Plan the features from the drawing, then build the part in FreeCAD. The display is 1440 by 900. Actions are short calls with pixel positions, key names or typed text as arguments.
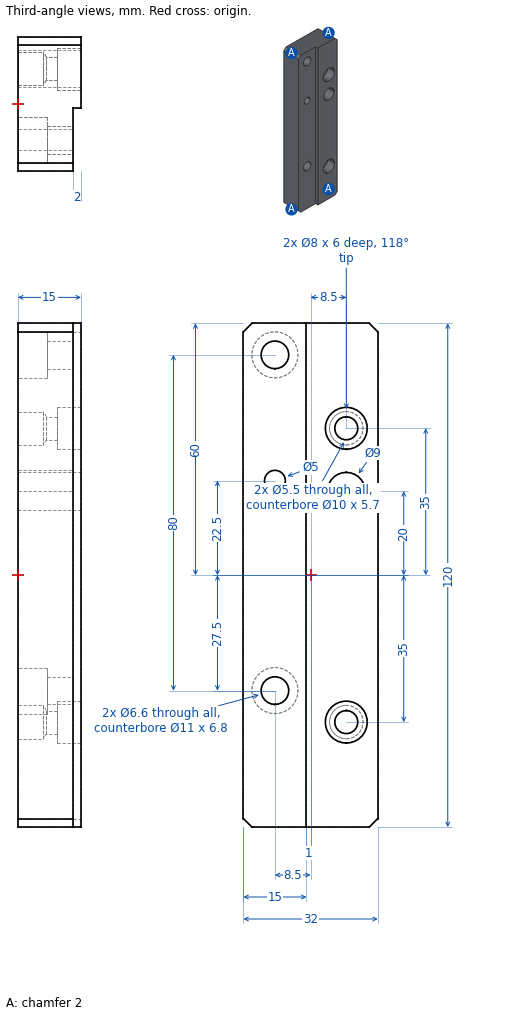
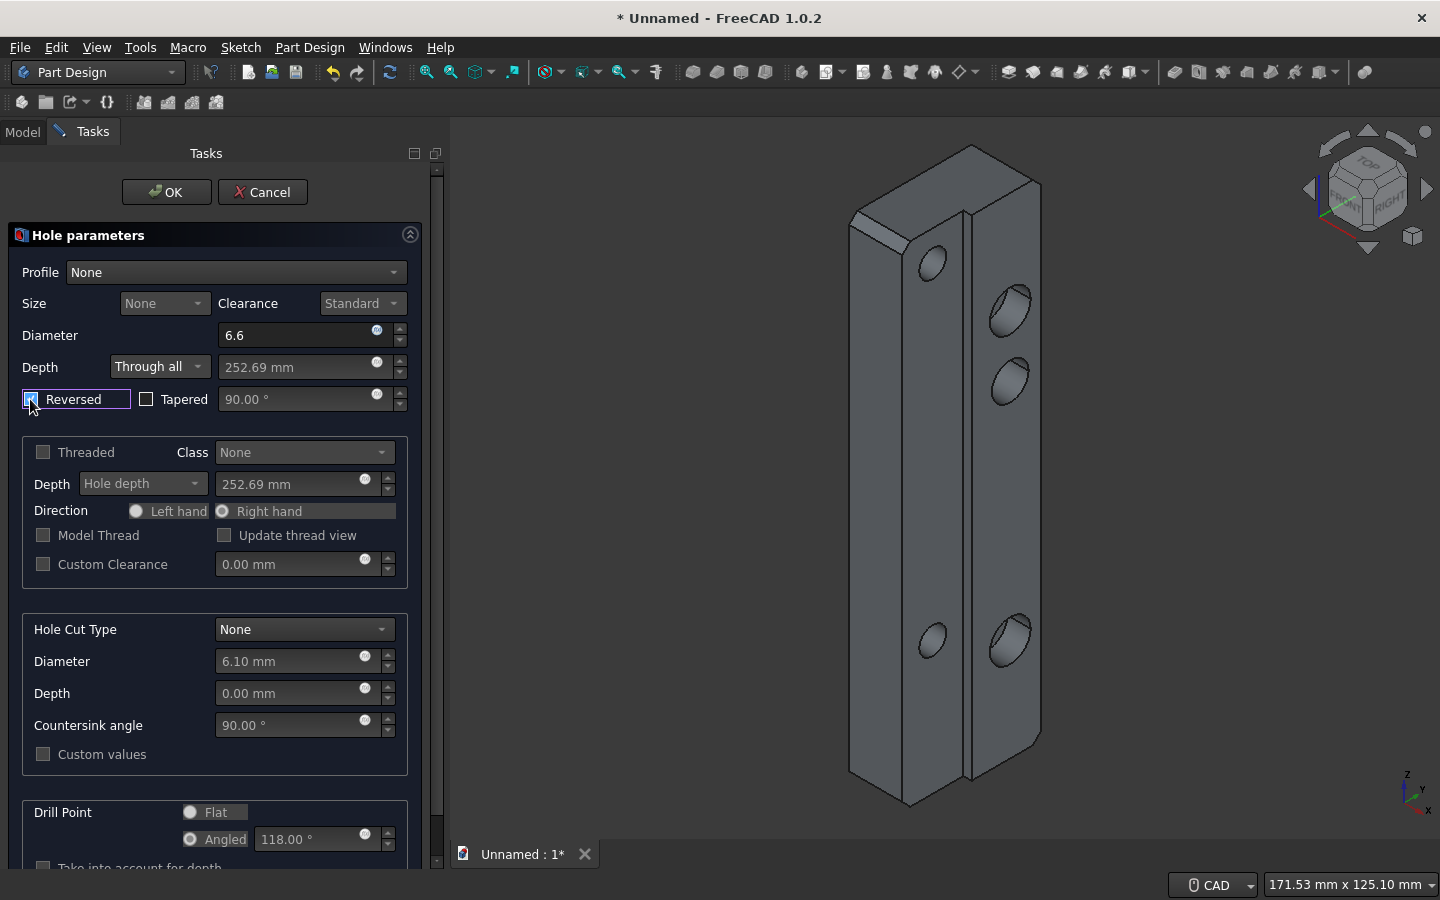
click(306, 630)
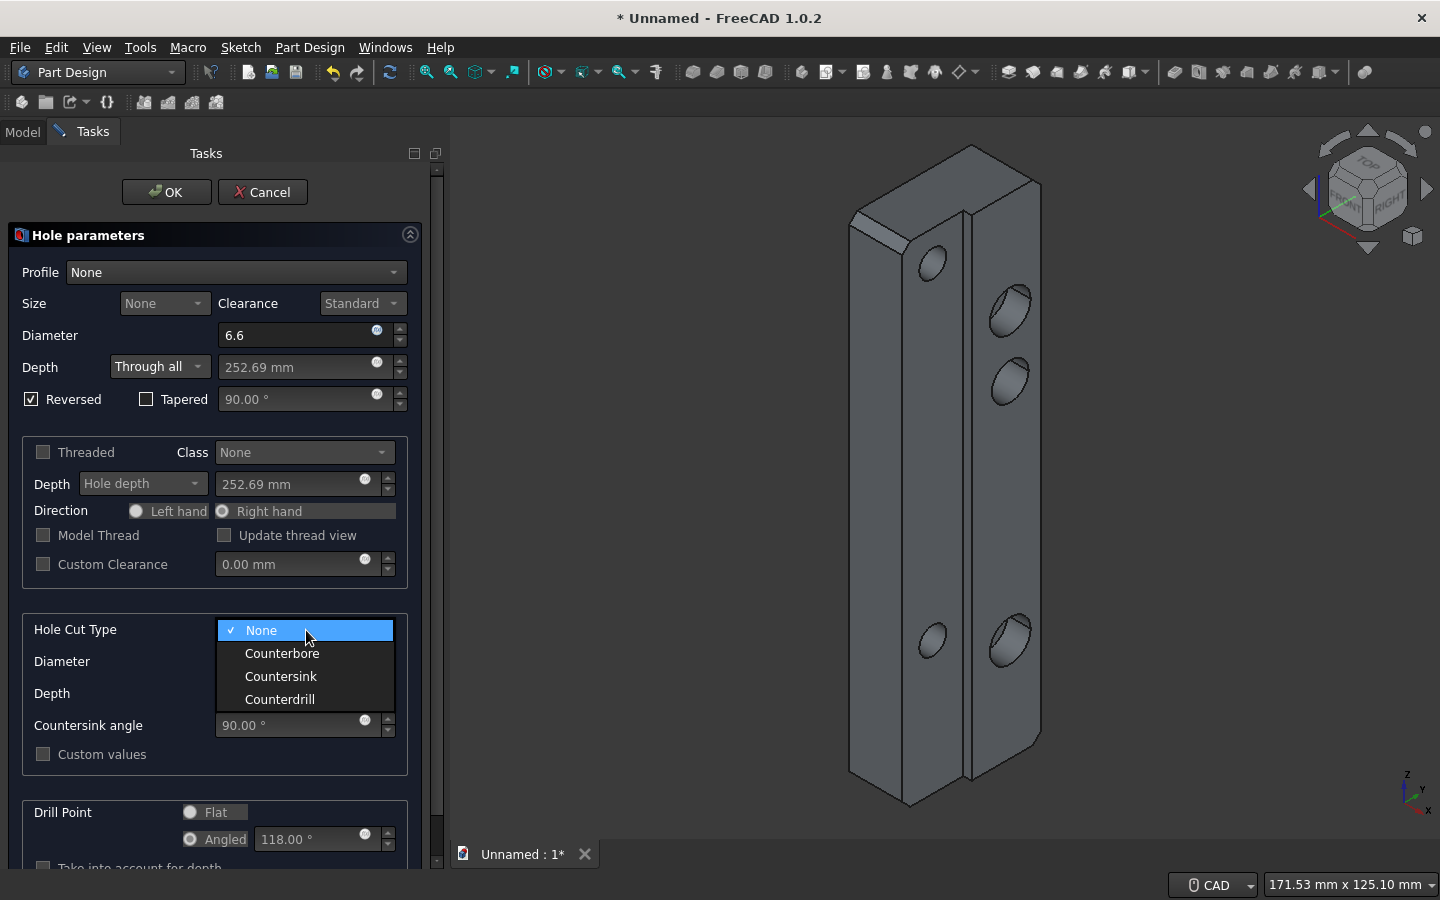
click(304, 654)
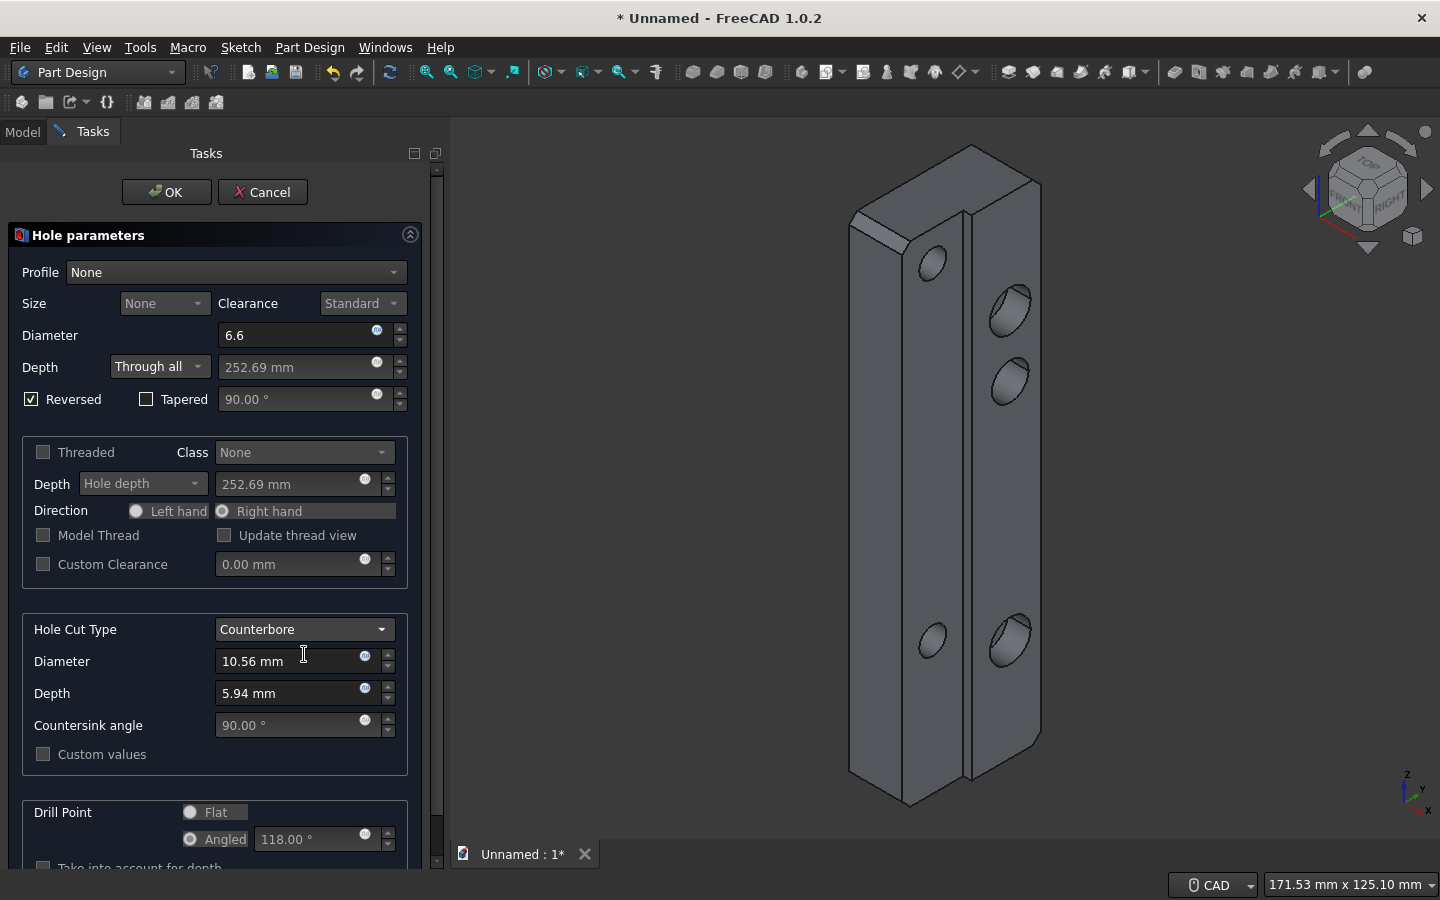
triple_click(298, 661)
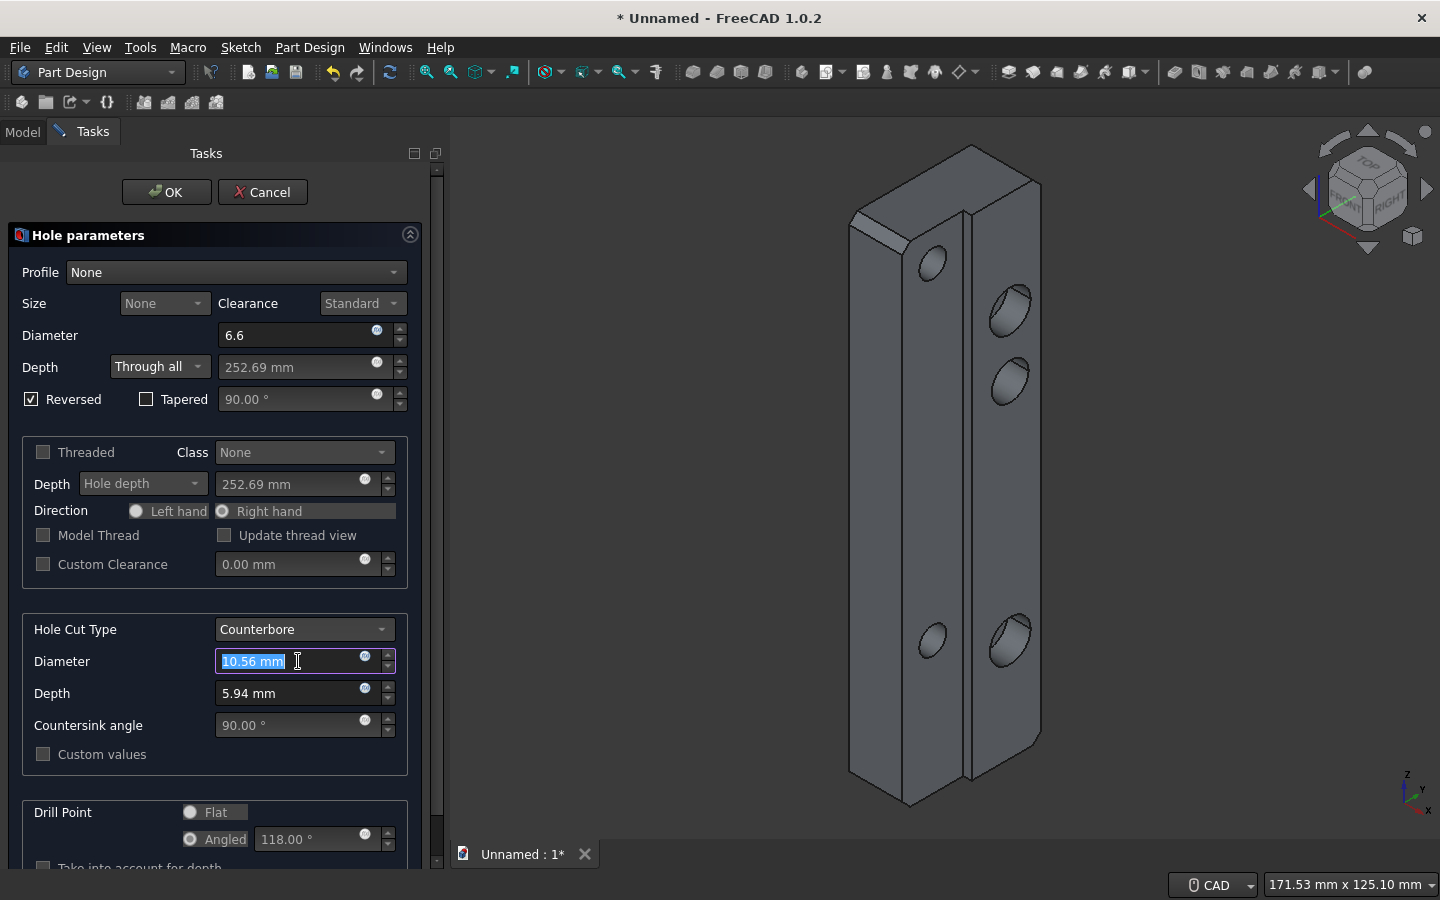
text(11)
key(Tab)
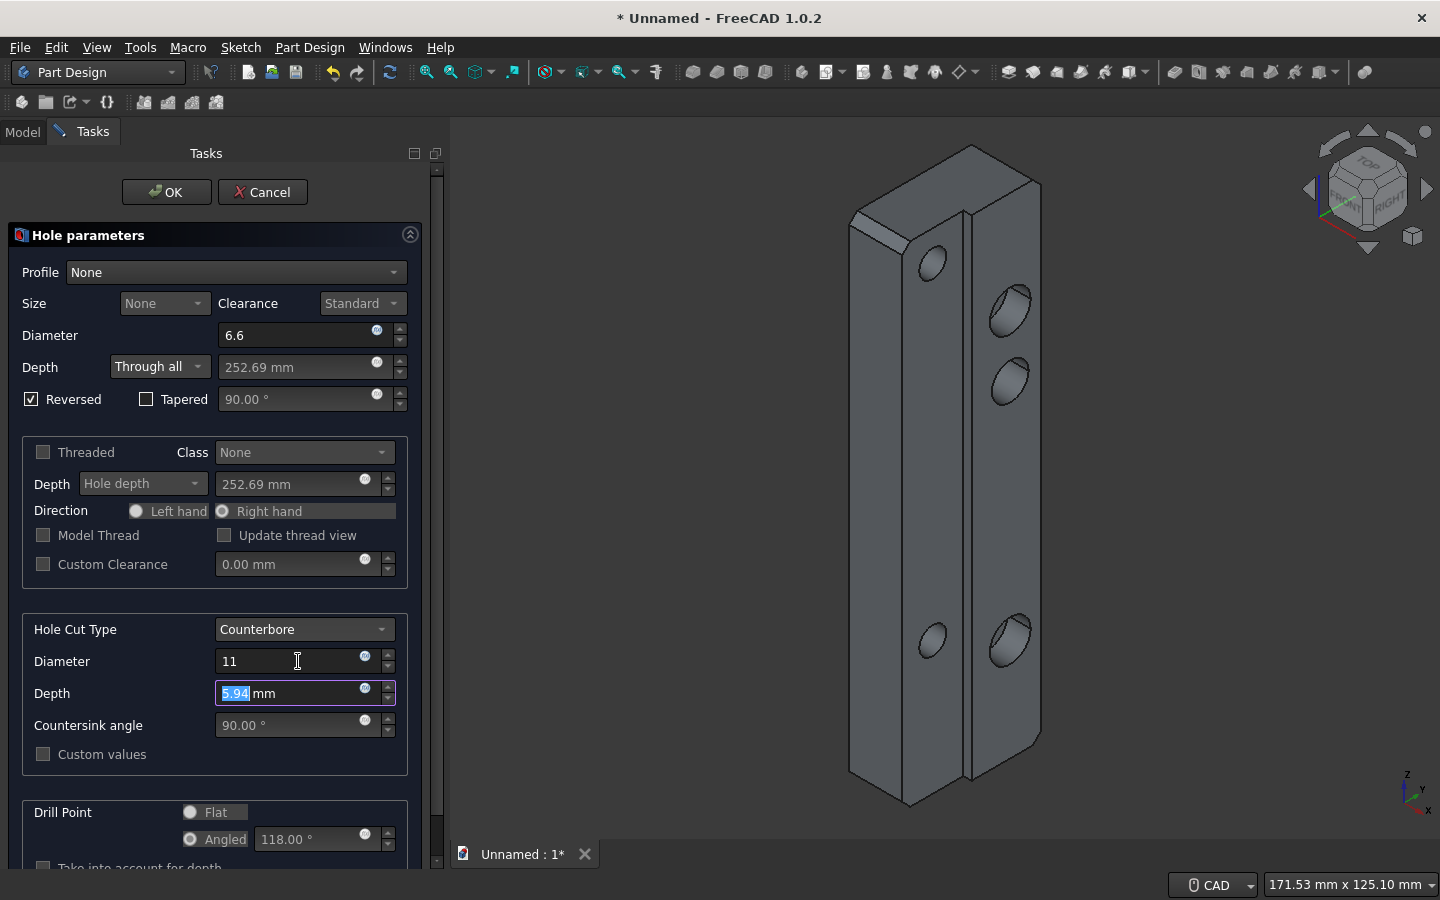
text(6.8)
key(Tab)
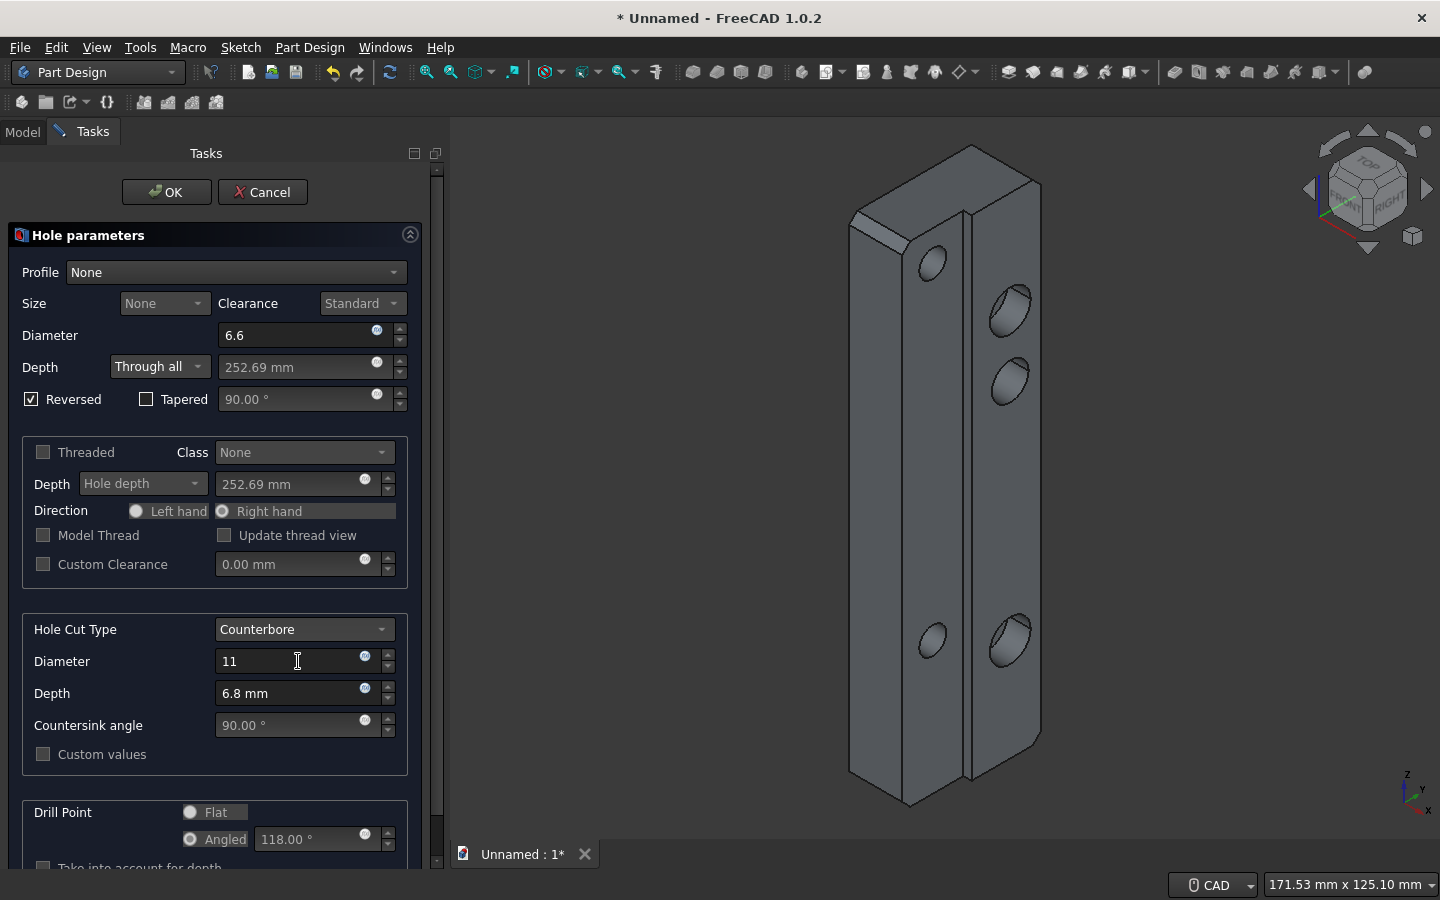
click(167, 192)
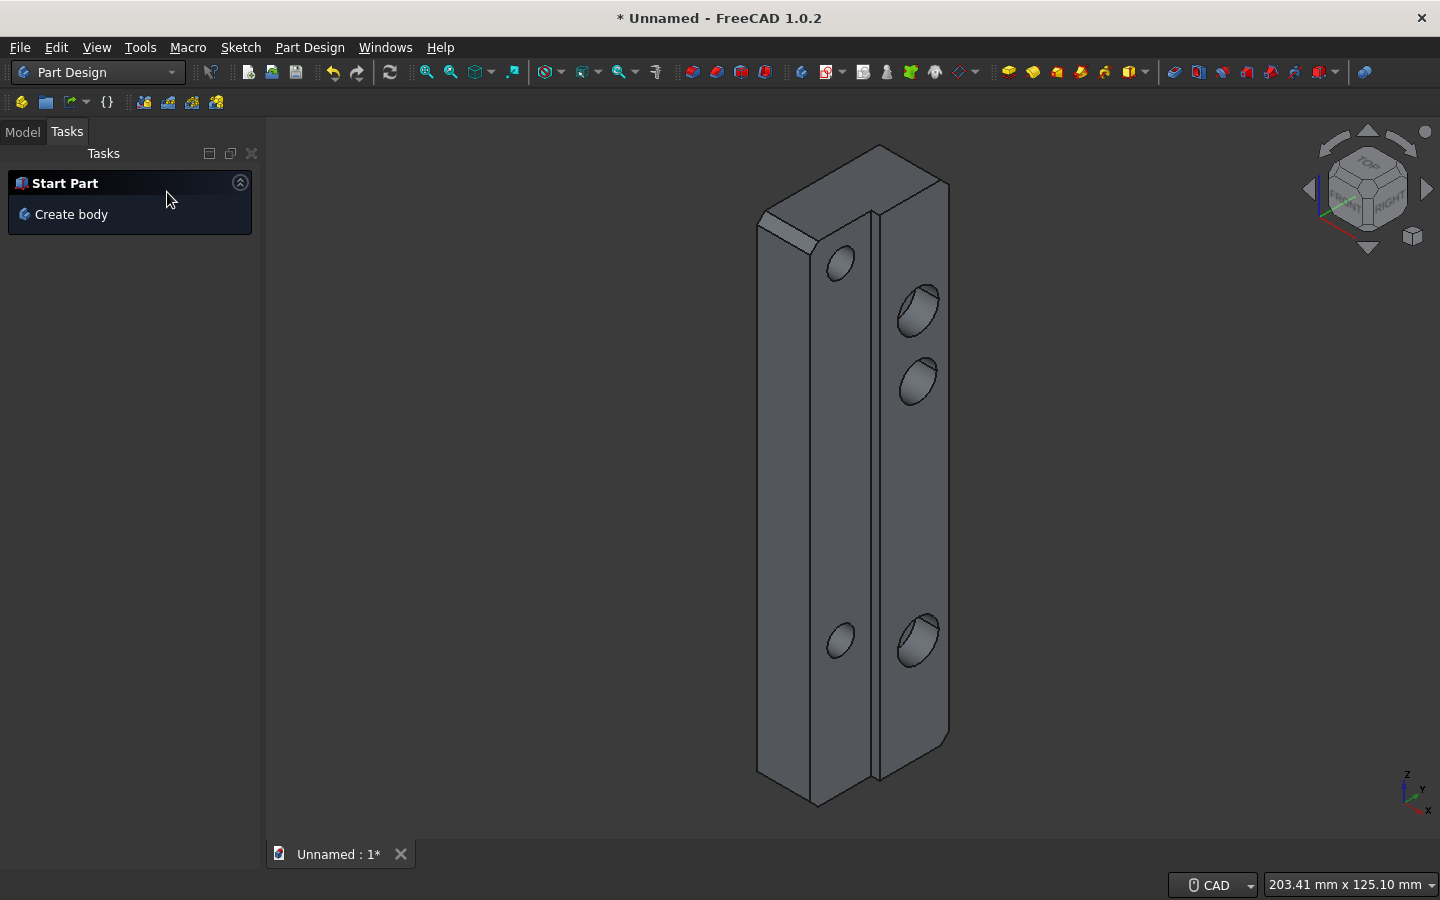
key(6)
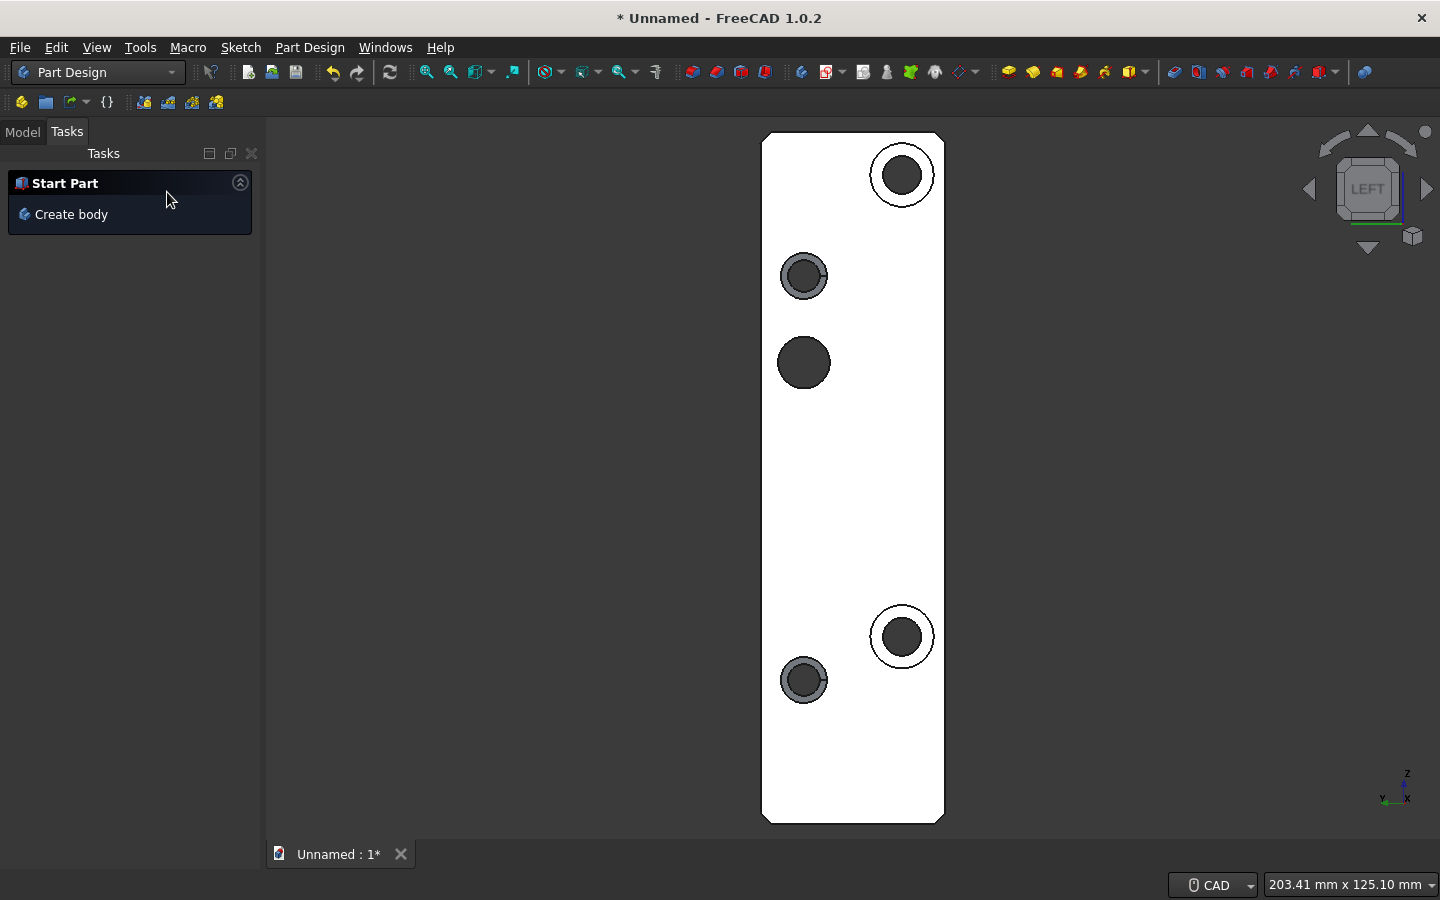
click(853, 477)